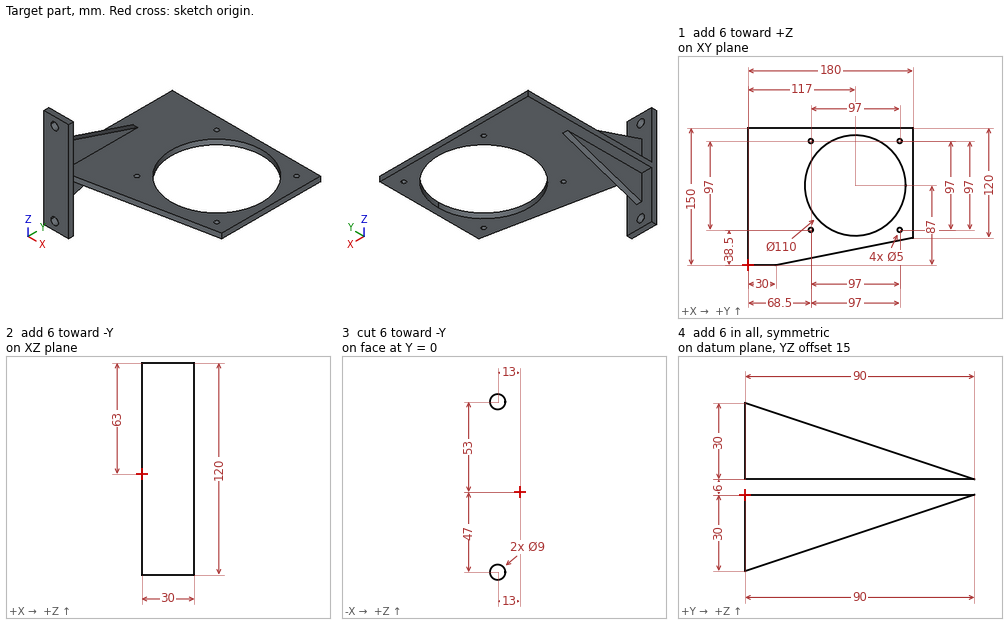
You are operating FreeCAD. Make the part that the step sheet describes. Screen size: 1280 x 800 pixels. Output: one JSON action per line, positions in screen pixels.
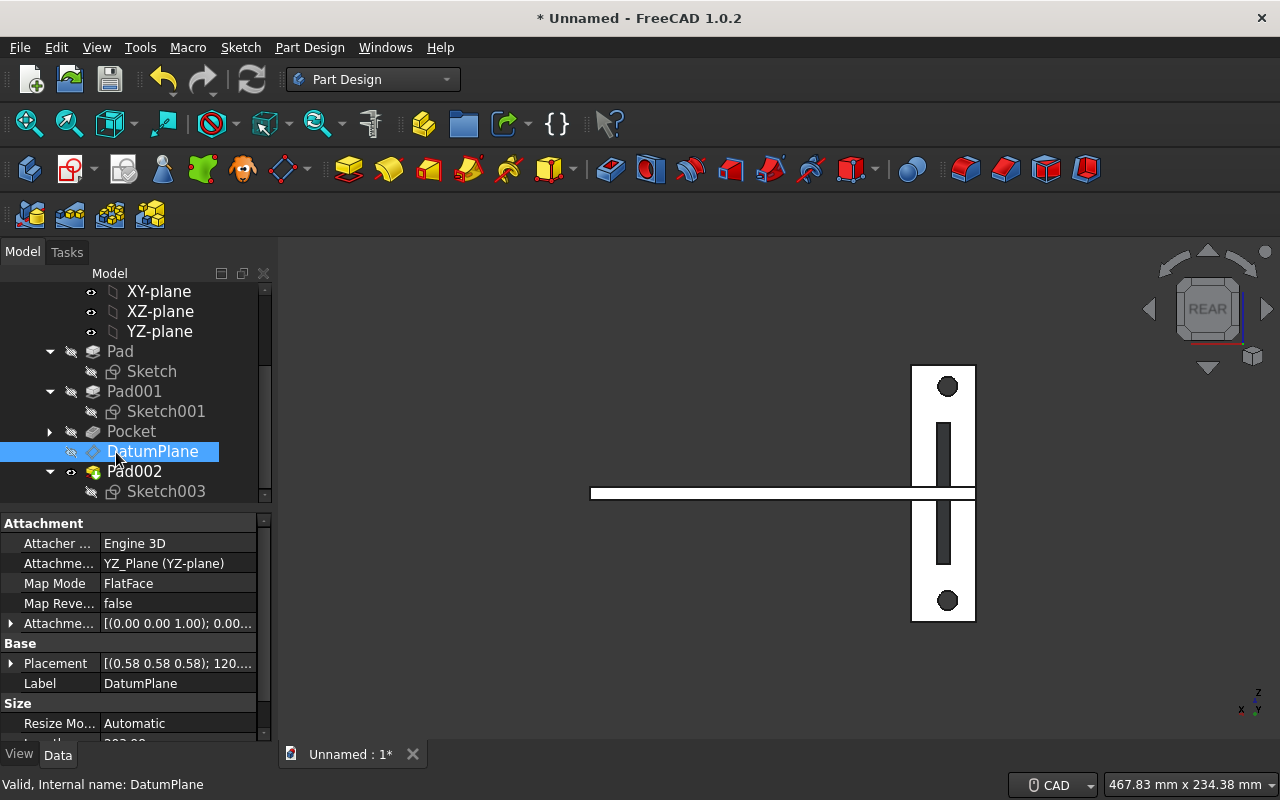
{"action": "key", "text": "0"}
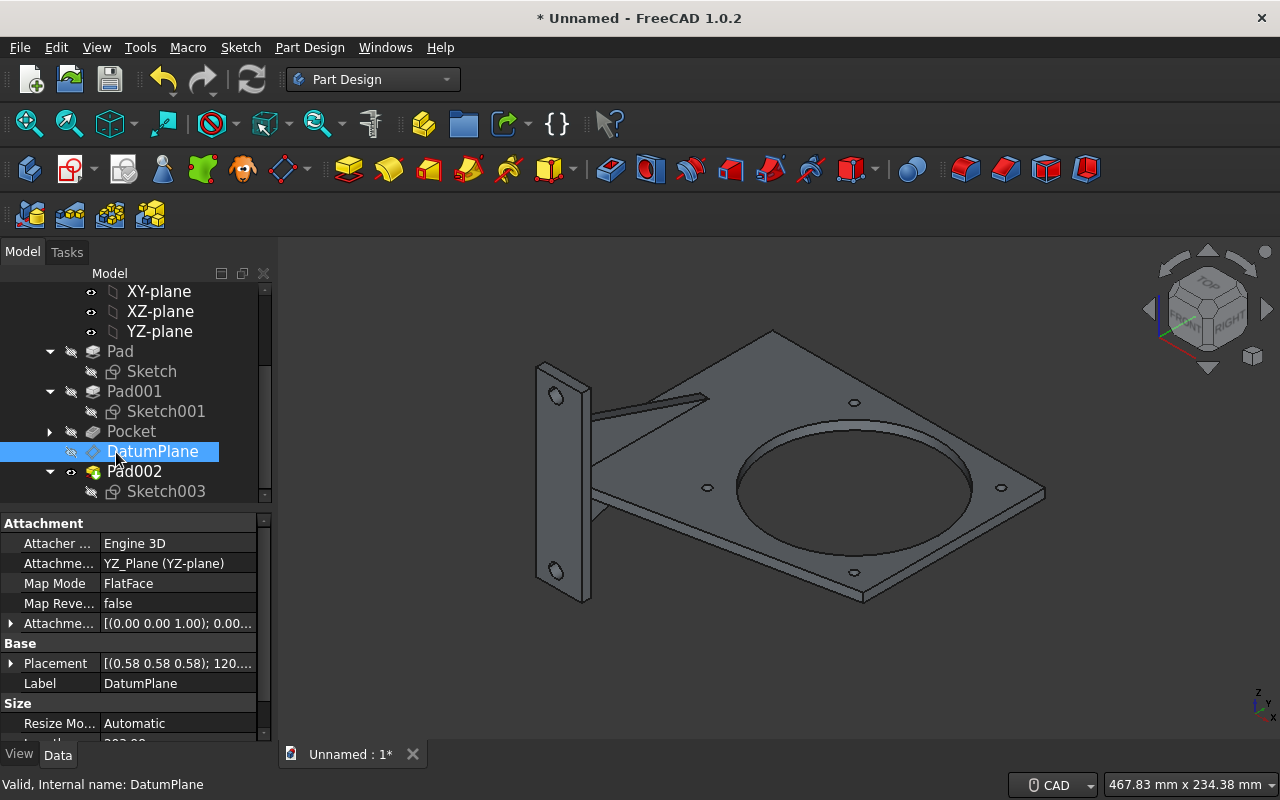
{"action": "key", "text": "v f"}